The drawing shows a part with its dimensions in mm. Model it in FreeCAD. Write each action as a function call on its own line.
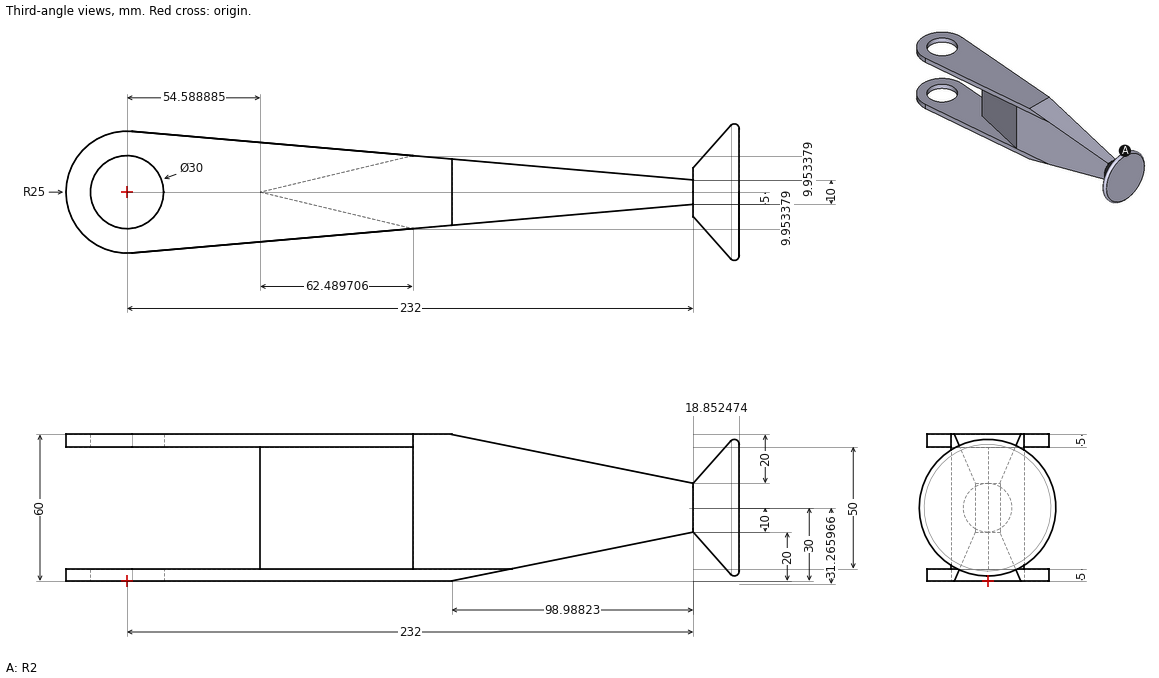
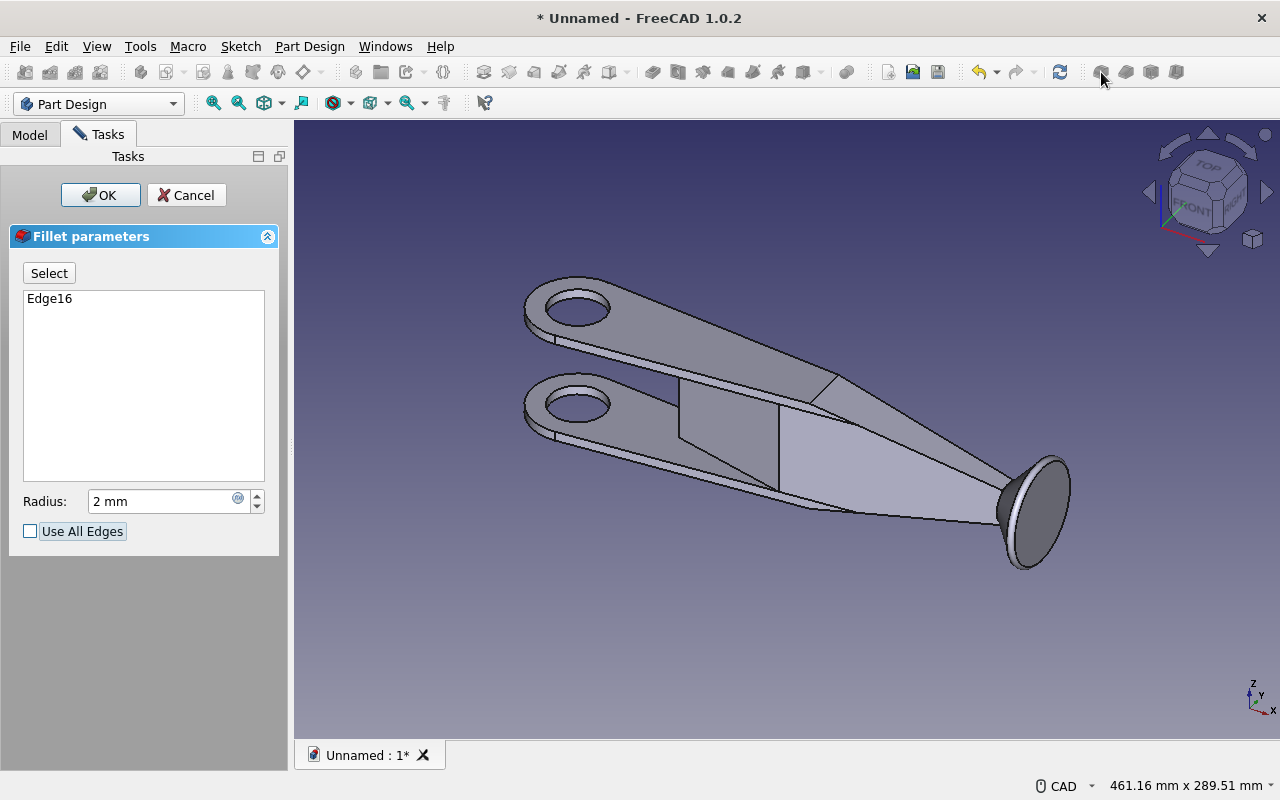
click(101, 195)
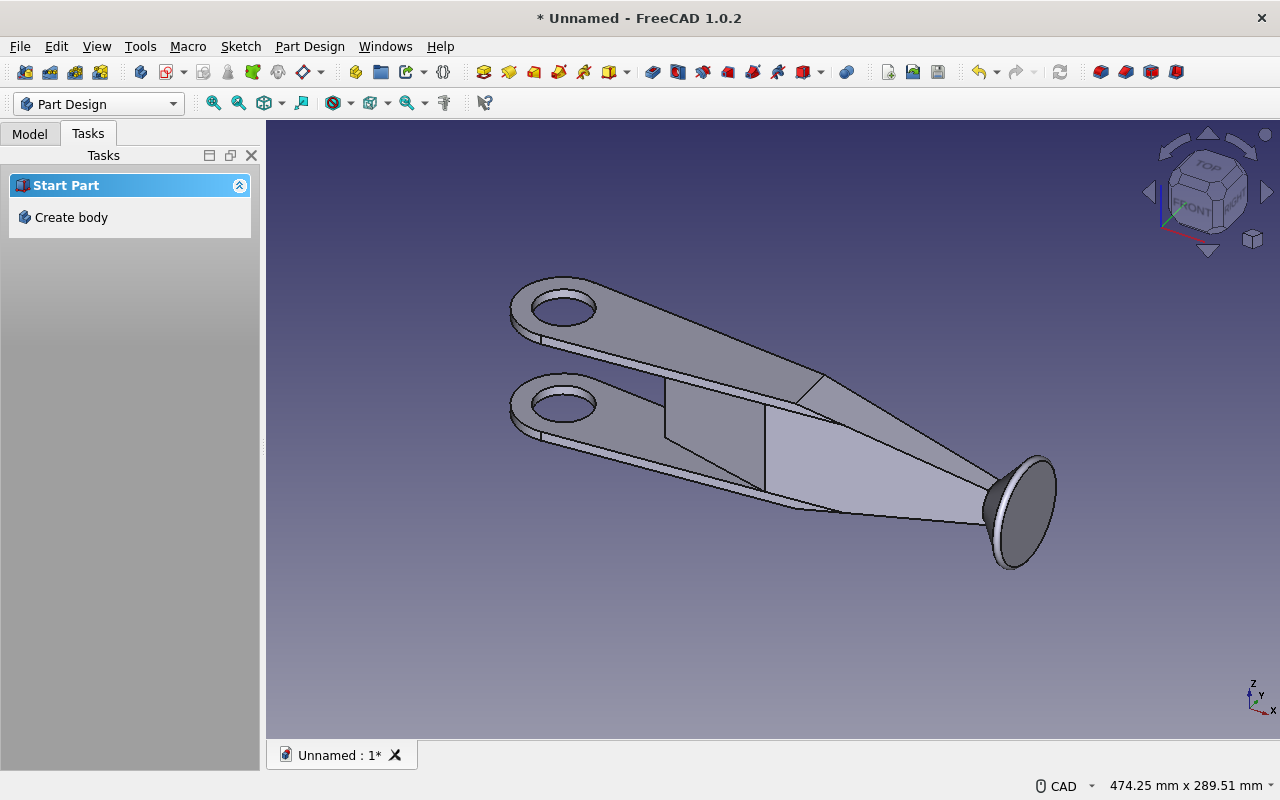
key(0)